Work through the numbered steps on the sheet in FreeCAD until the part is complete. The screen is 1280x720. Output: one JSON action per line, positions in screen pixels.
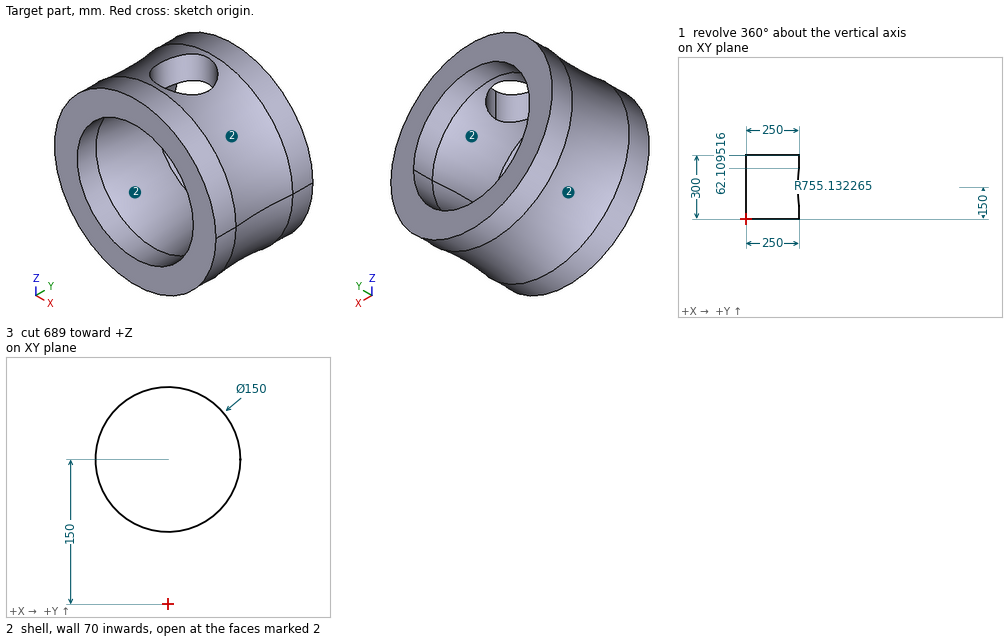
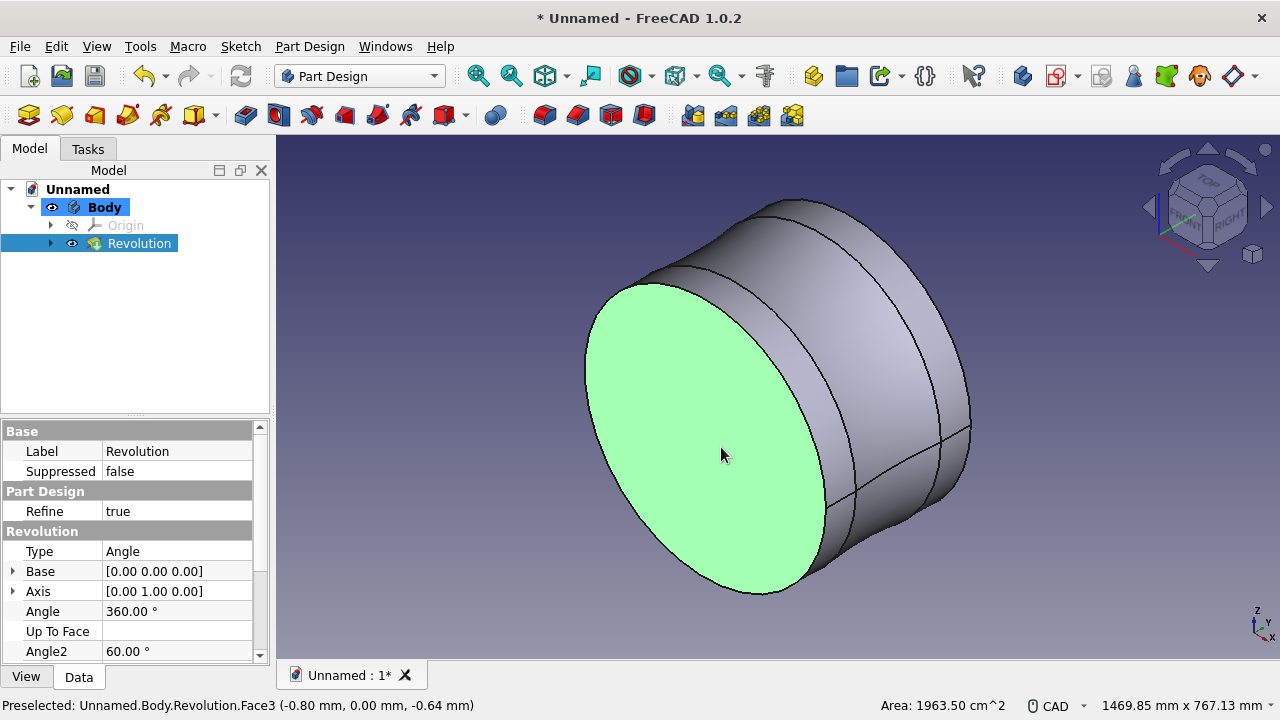
{"action": "key", "text": "2"}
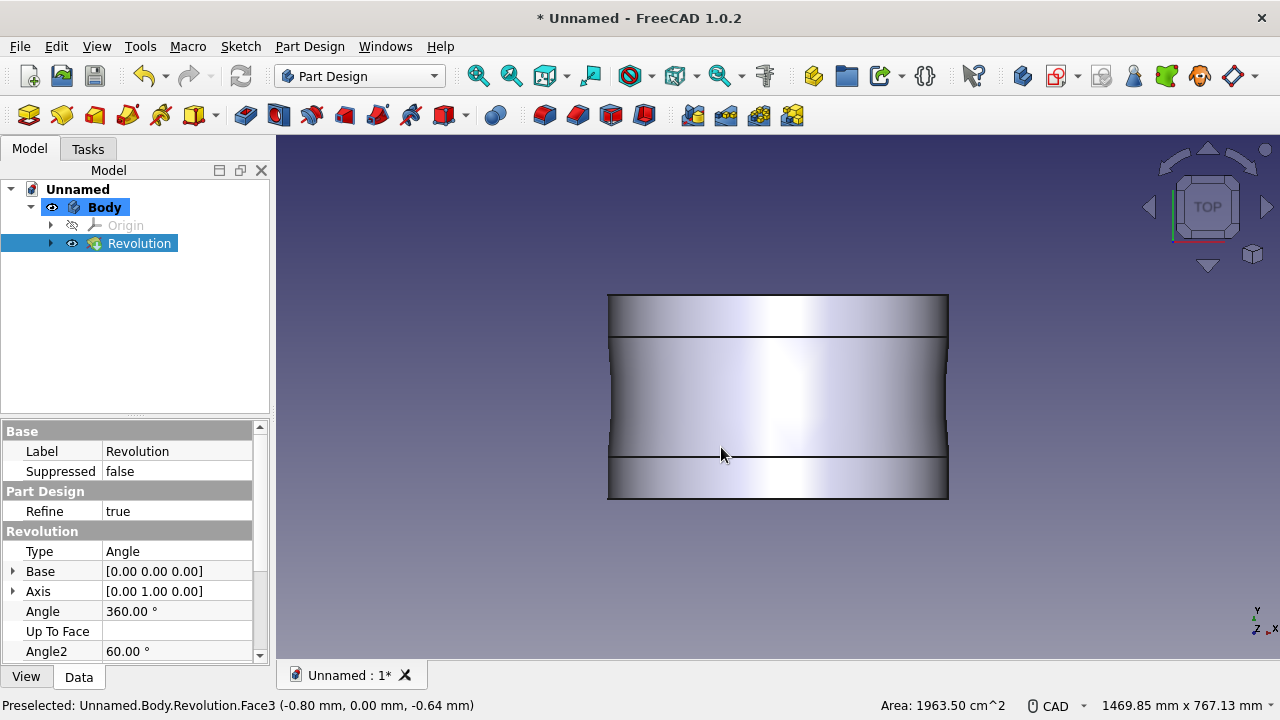
{"action": "left_click", "coordinate": [479, 76]}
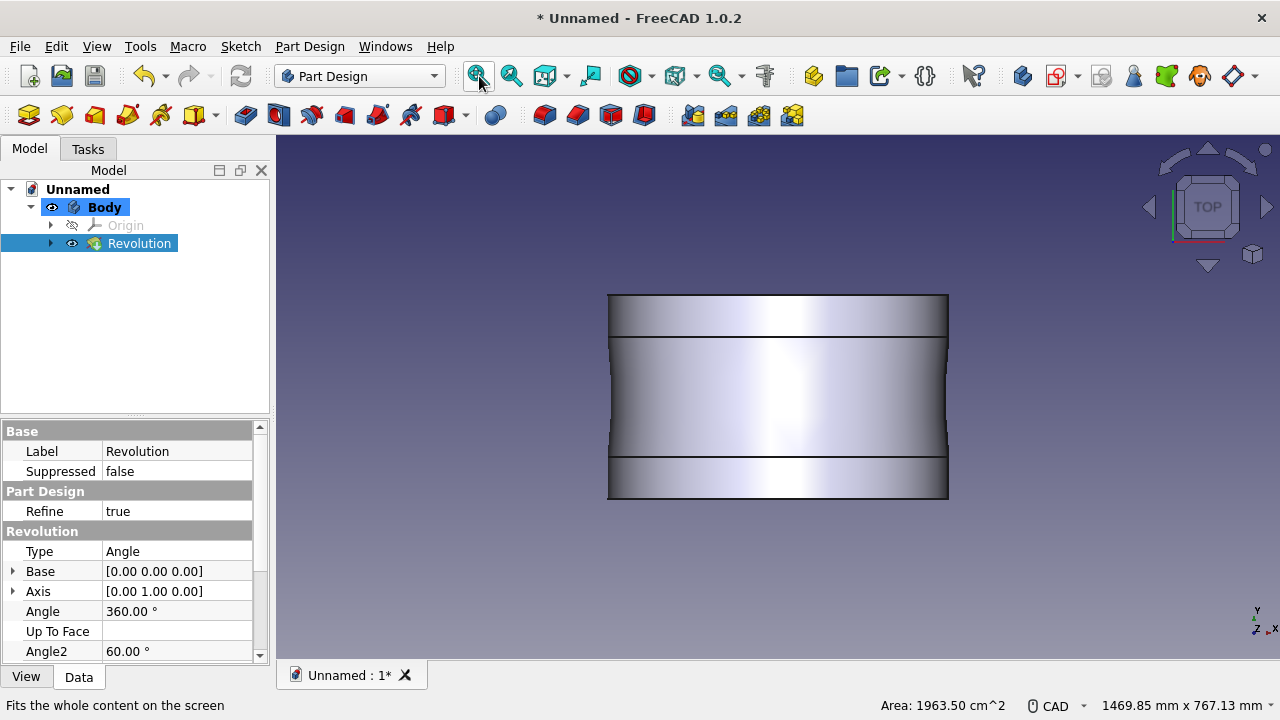
{"action": "key", "text": "1"}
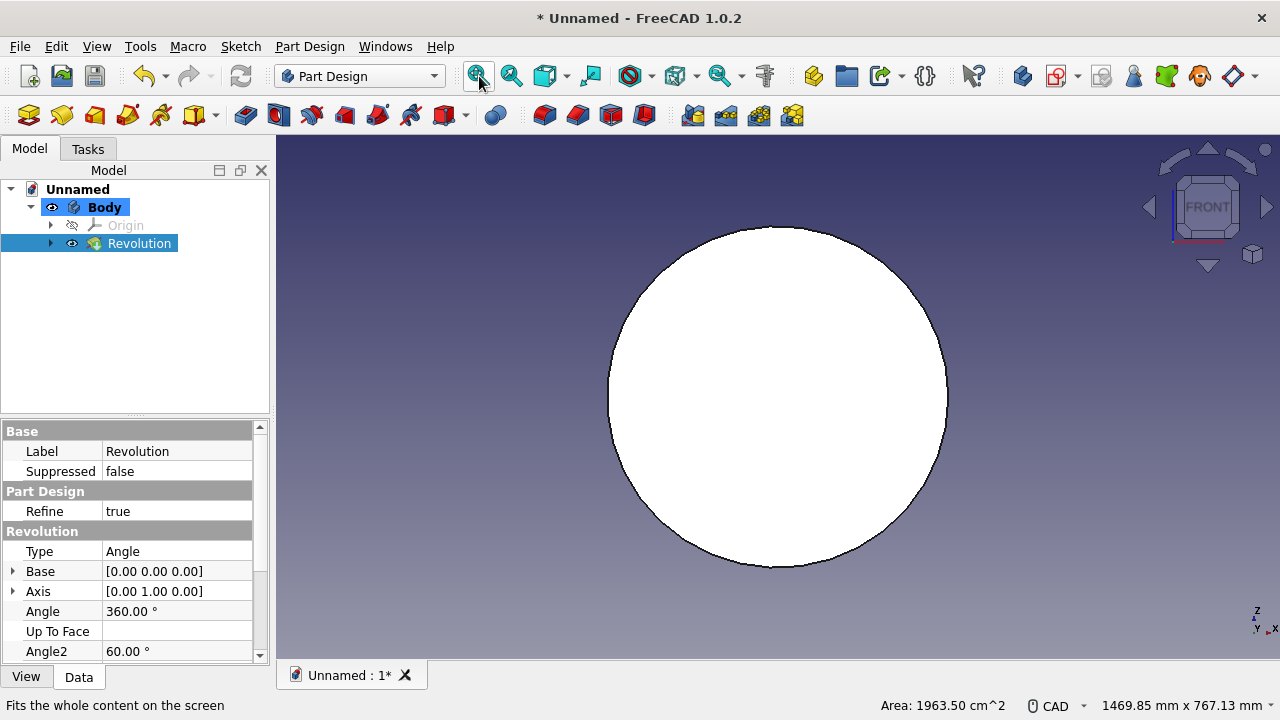
{"action": "key", "text": "3"}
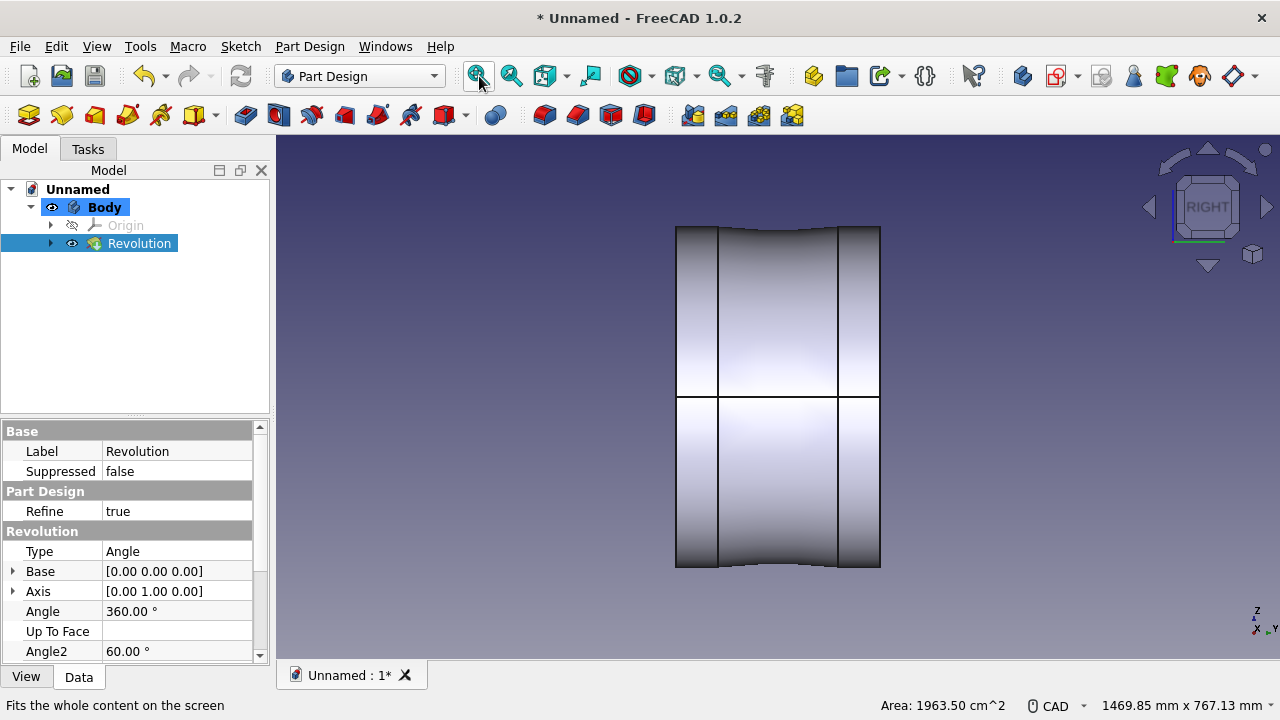
{"action": "key", "text": "5"}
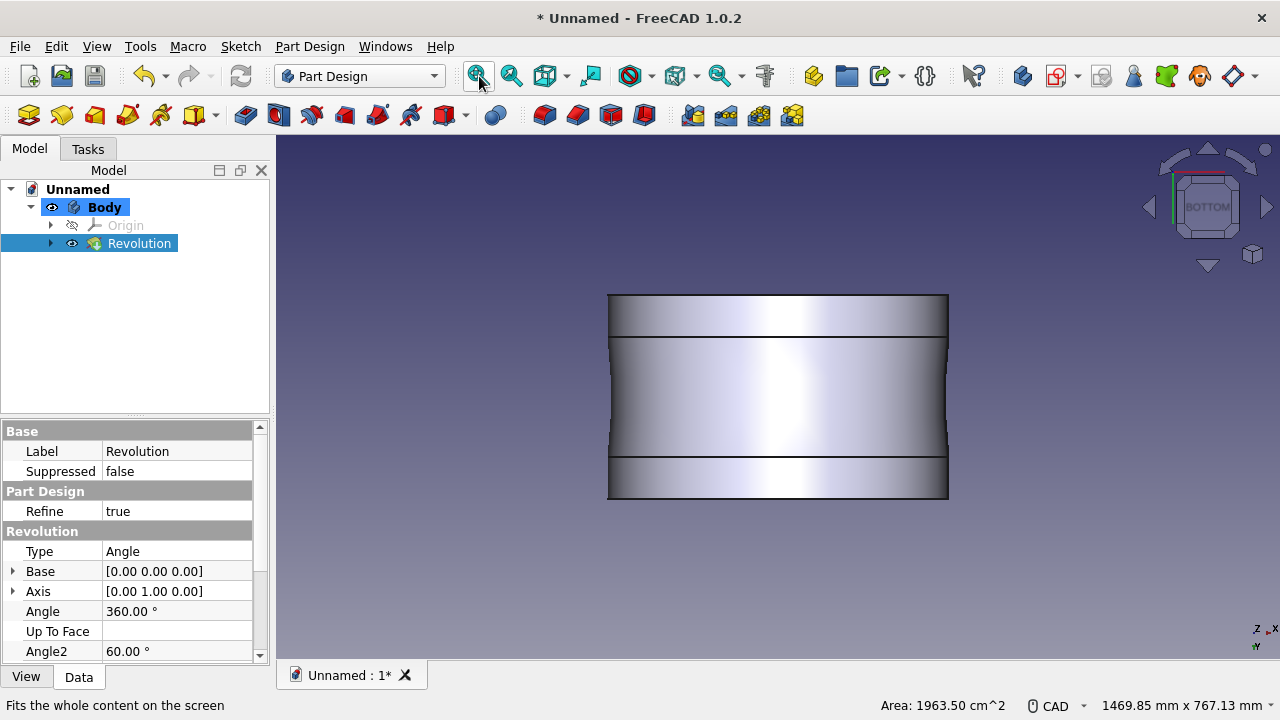
{"action": "left_click", "coordinate": [479, 76]}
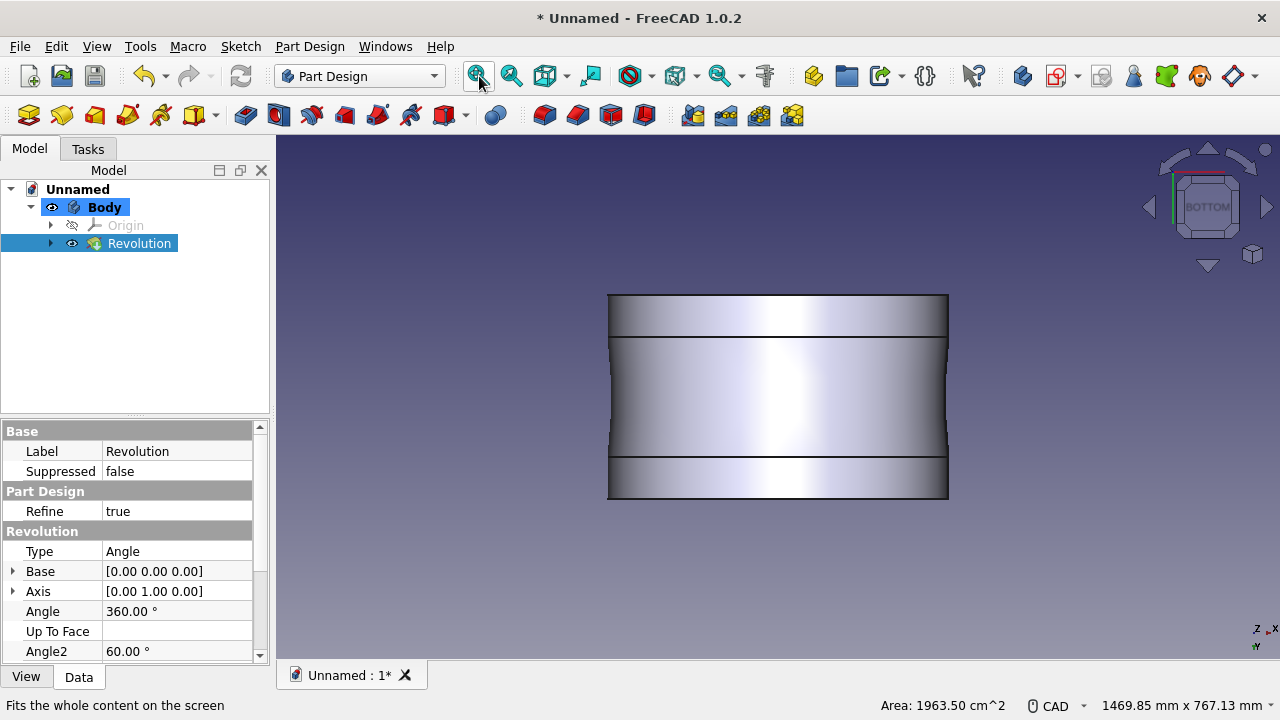
{"action": "key", "text": "4"}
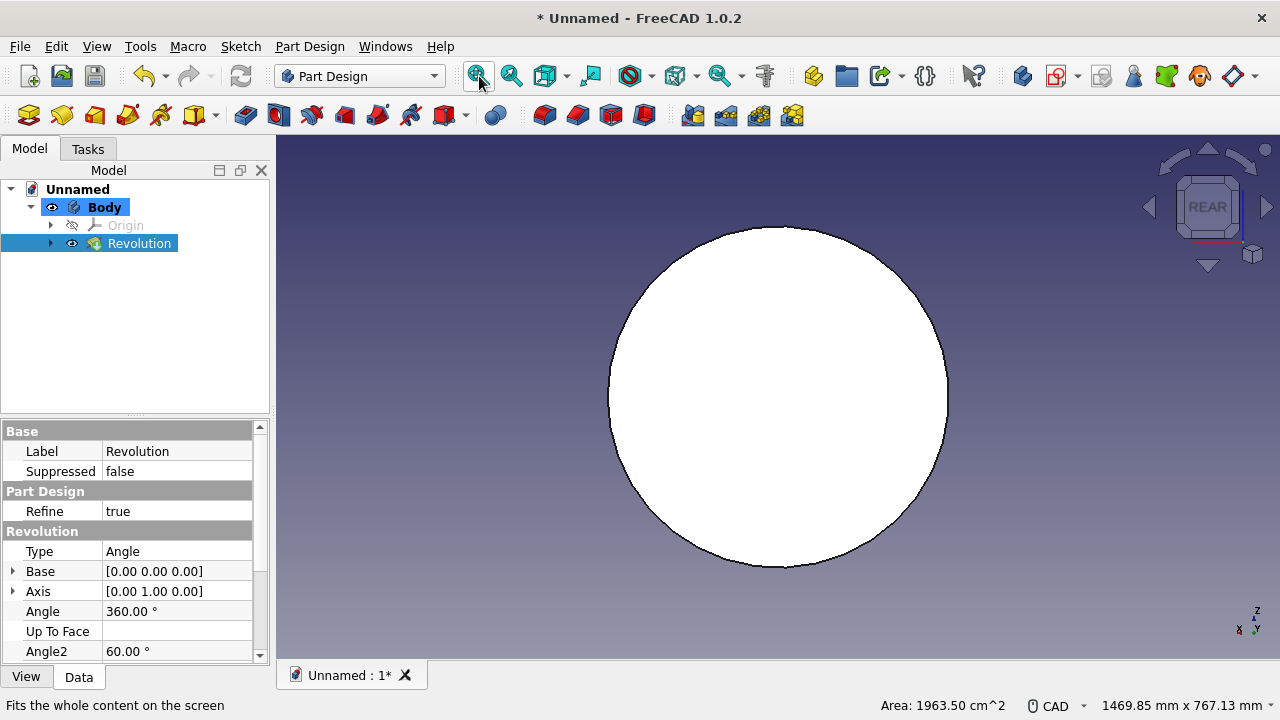
{"action": "left_click", "coordinate": [778, 396], "text": "ctrl"}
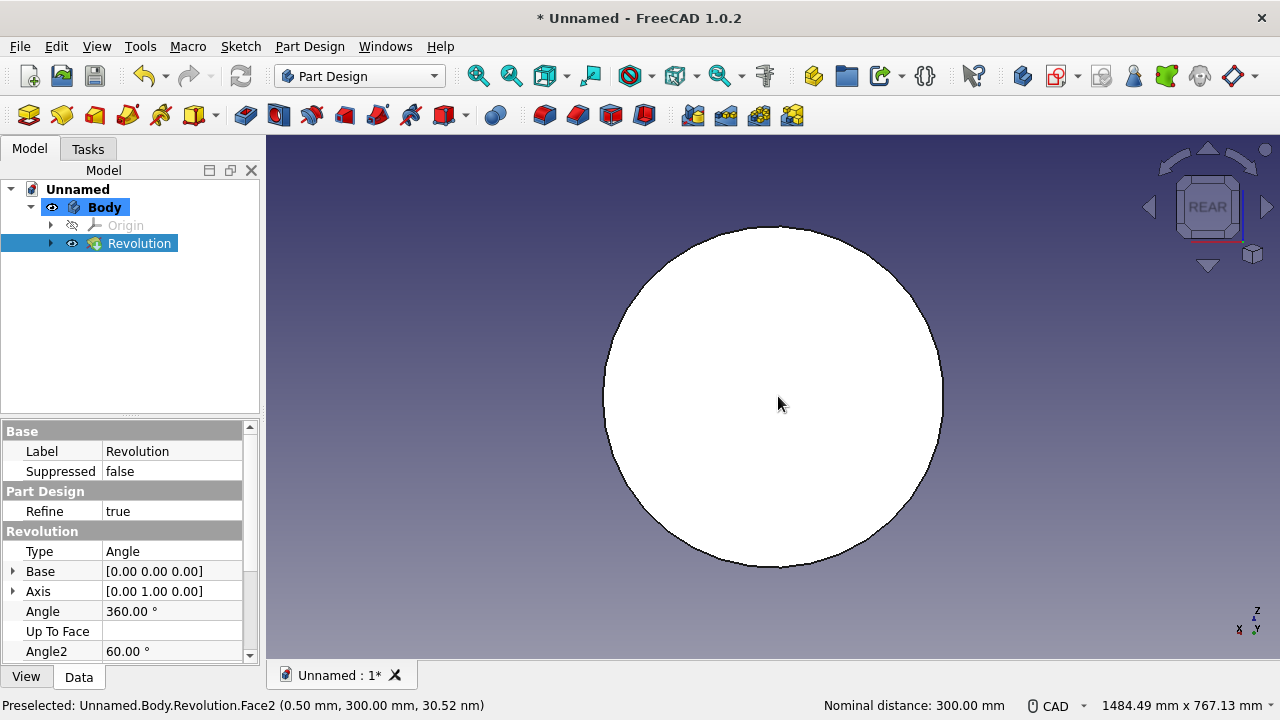
{"action": "left_click", "coordinate": [644, 116]}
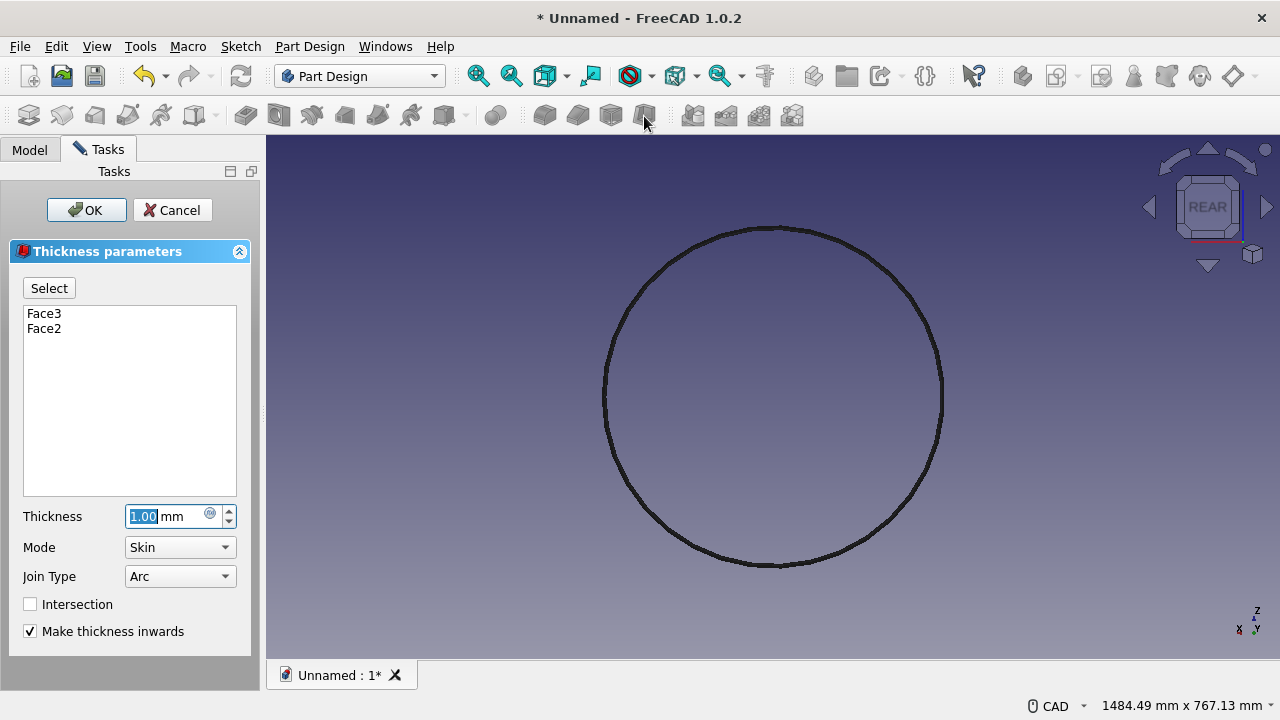
{"action": "type", "text": "70"}
{"action": "key", "text": "Tab"}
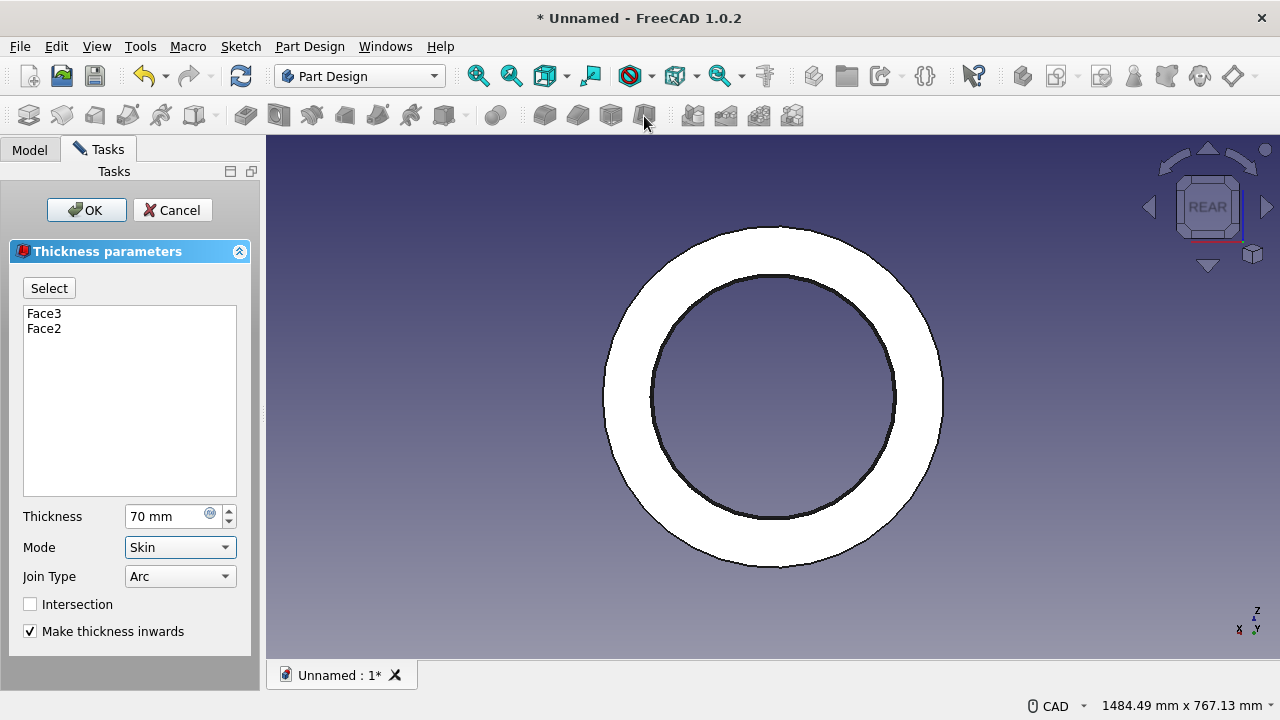
{"action": "left_click", "coordinate": [181, 576]}